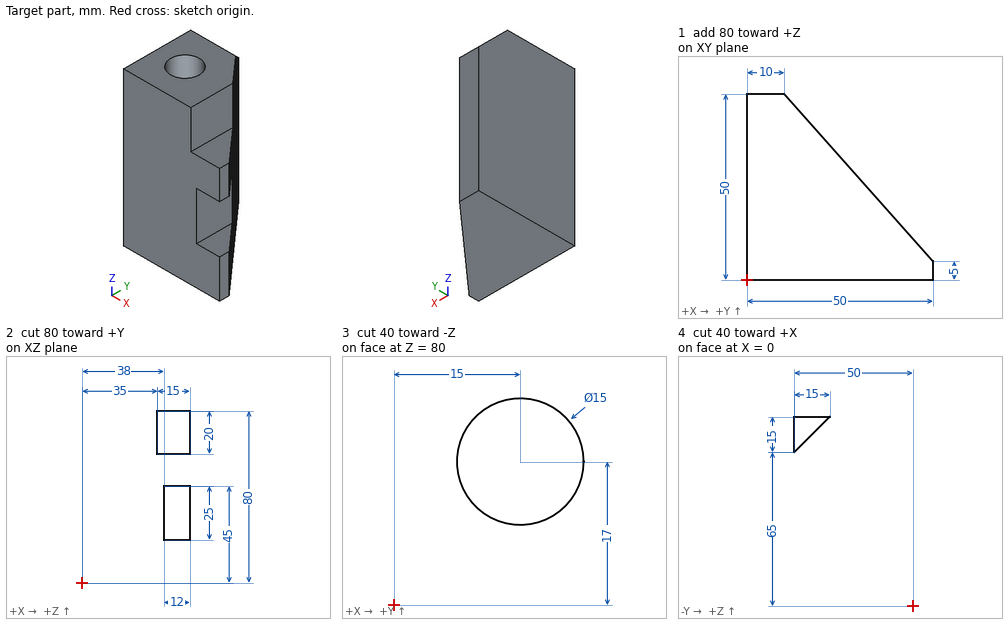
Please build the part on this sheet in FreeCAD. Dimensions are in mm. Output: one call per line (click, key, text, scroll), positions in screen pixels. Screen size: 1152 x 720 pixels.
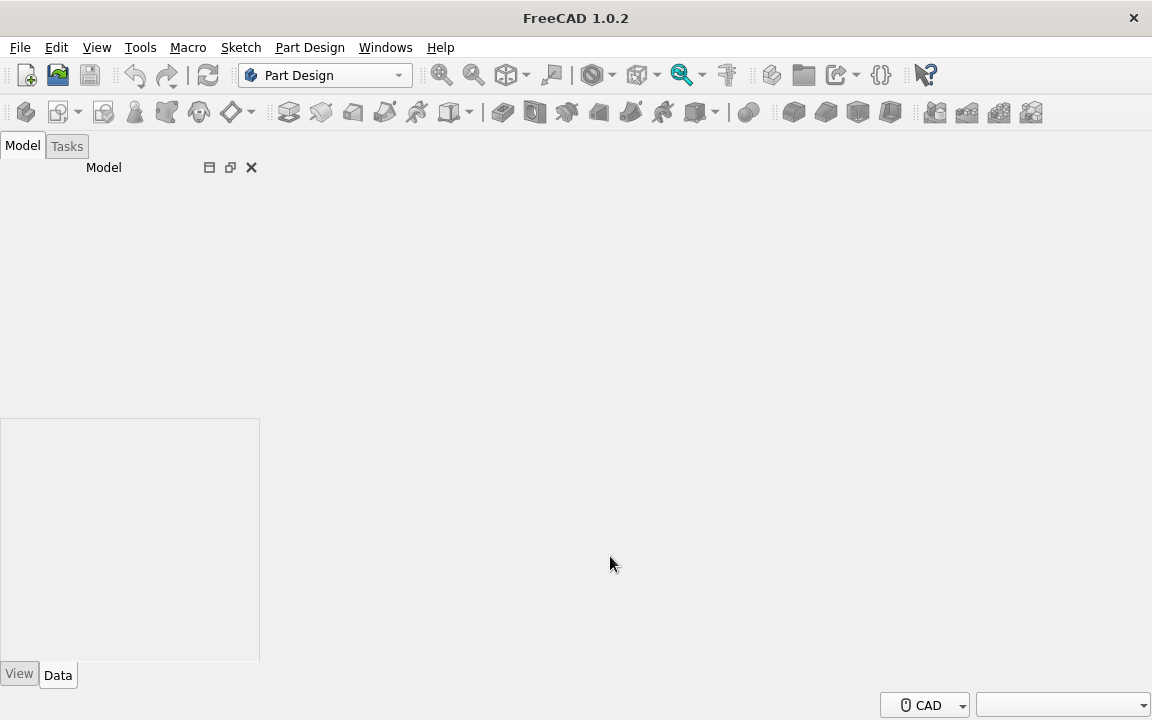
key(ctrl+n)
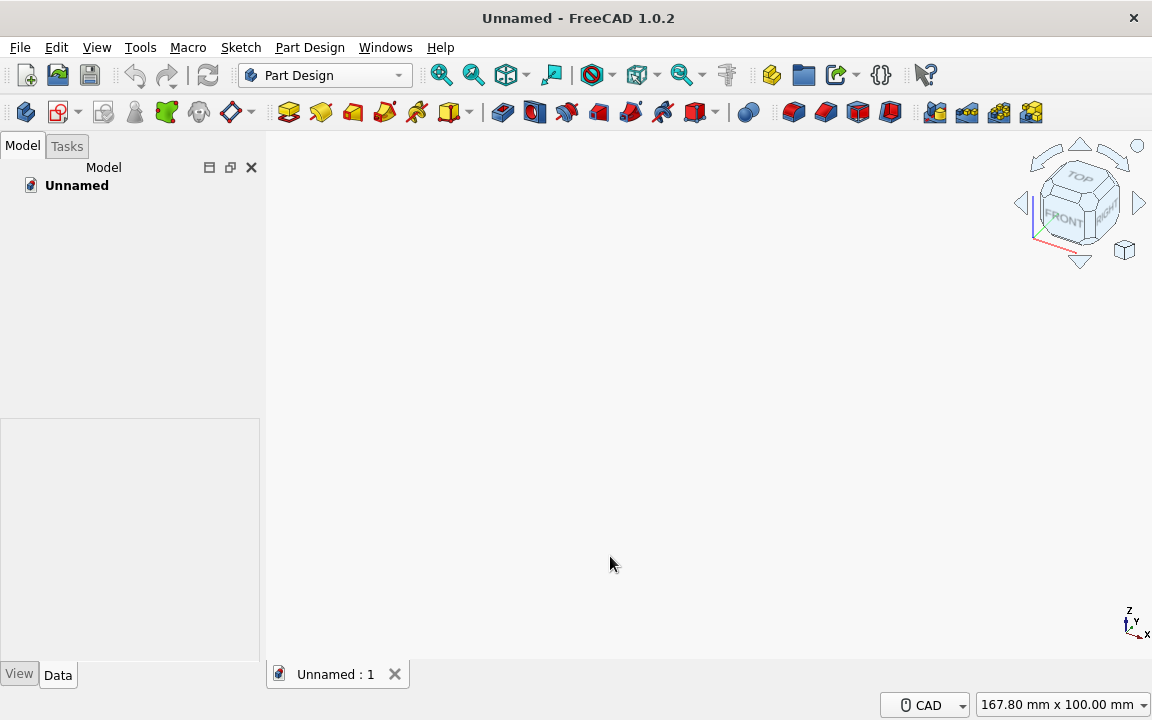
click(58, 112)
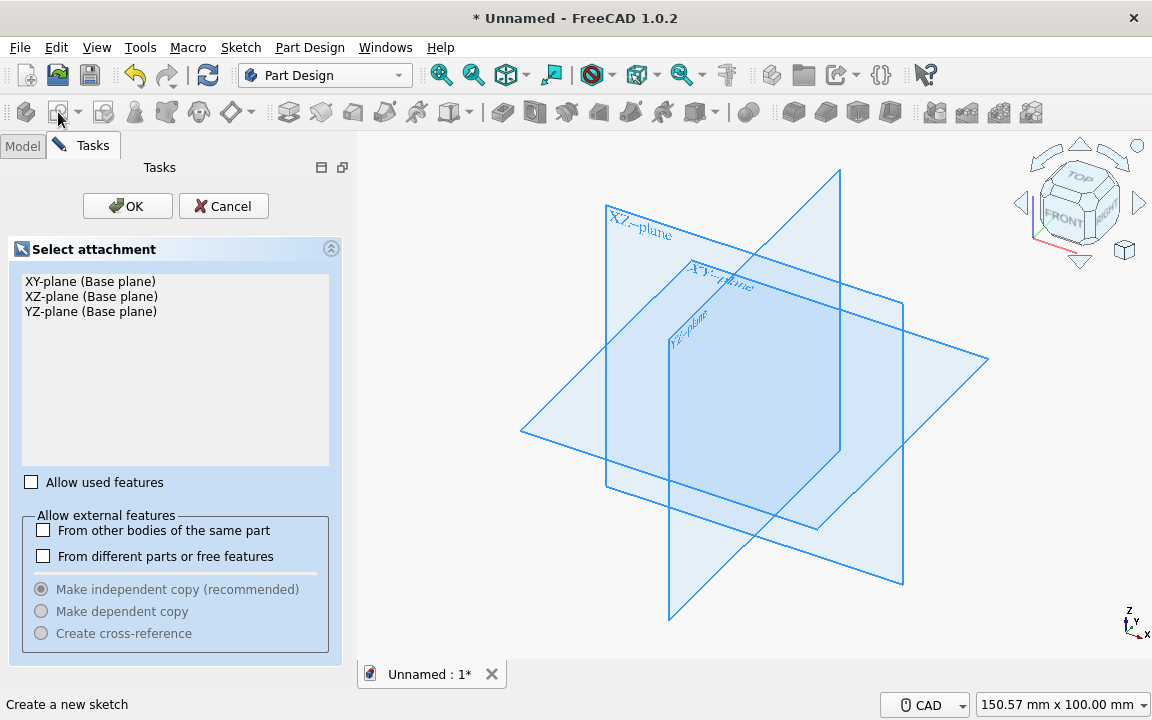
click(82, 282)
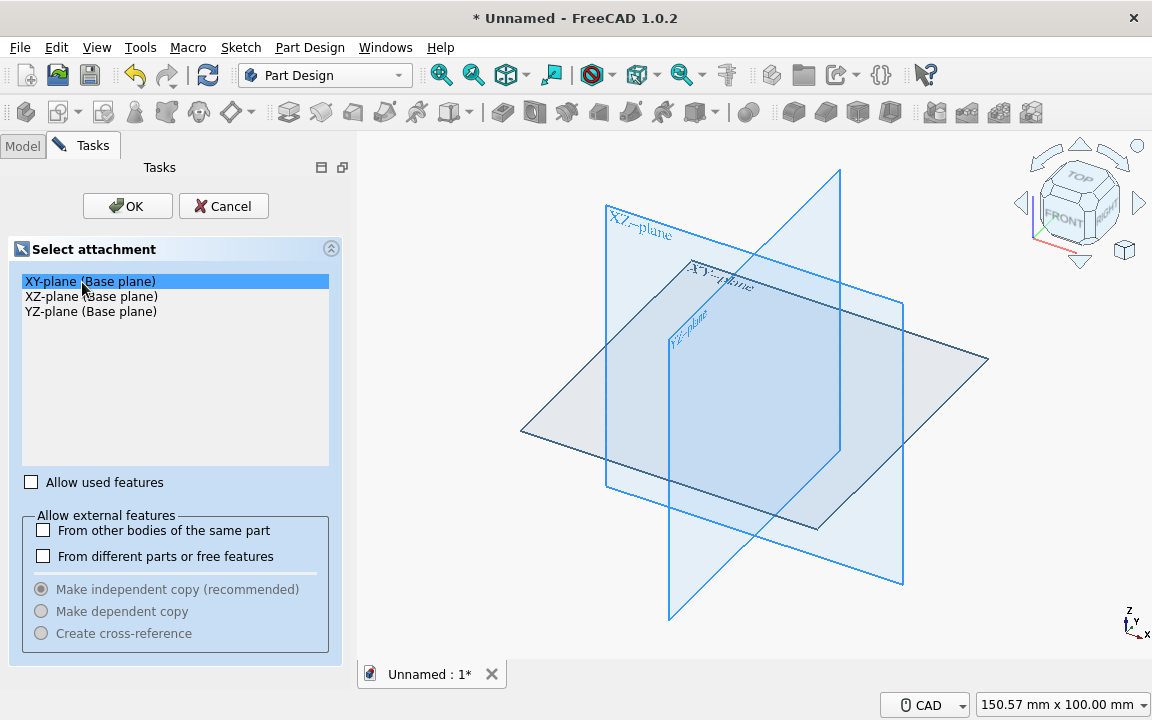
click(128, 206)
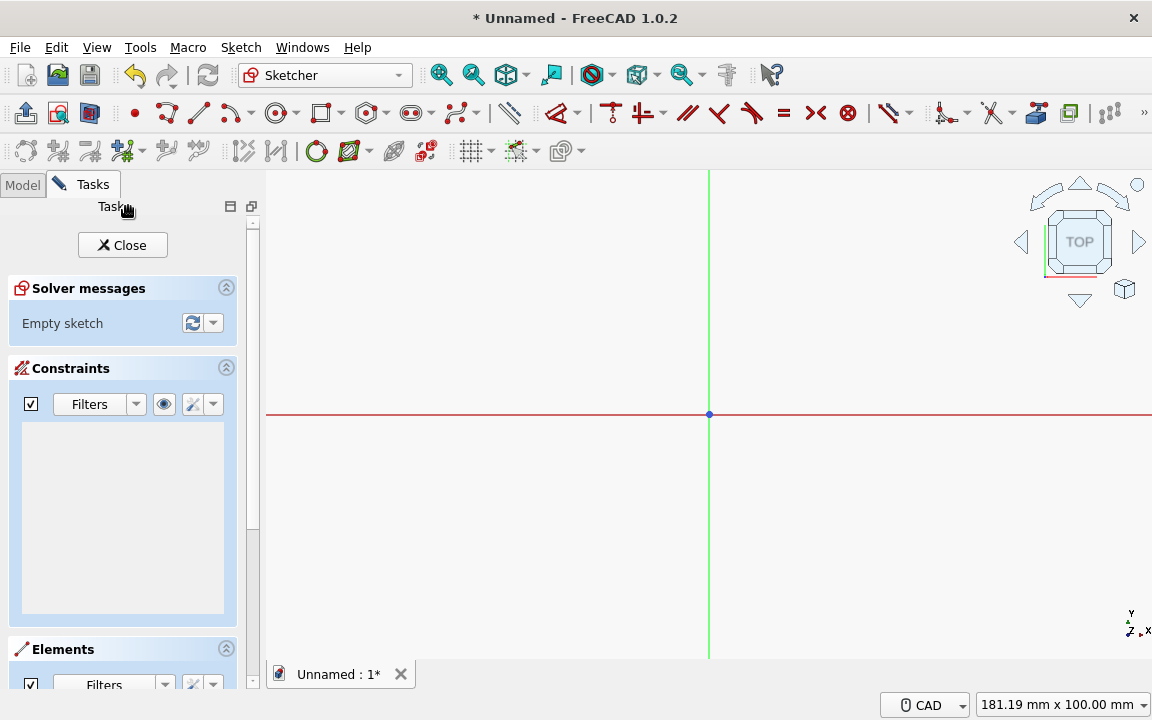
scroll(294, 631, down, 1)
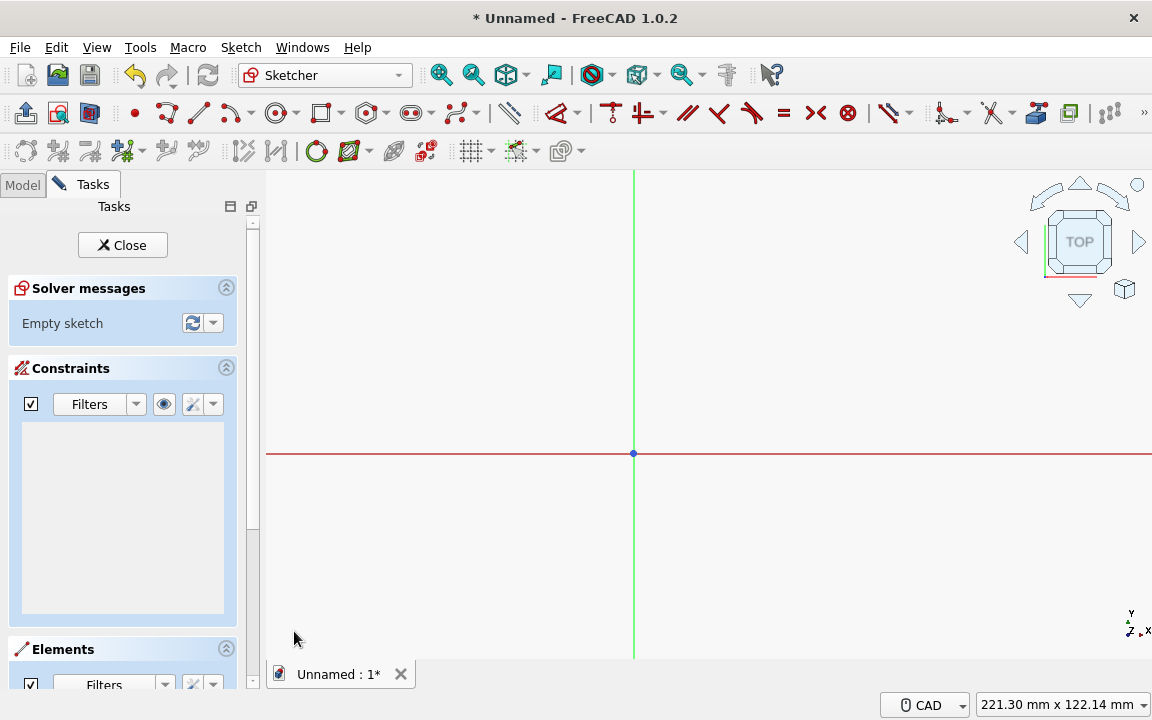
scroll(924, 230, up, 2)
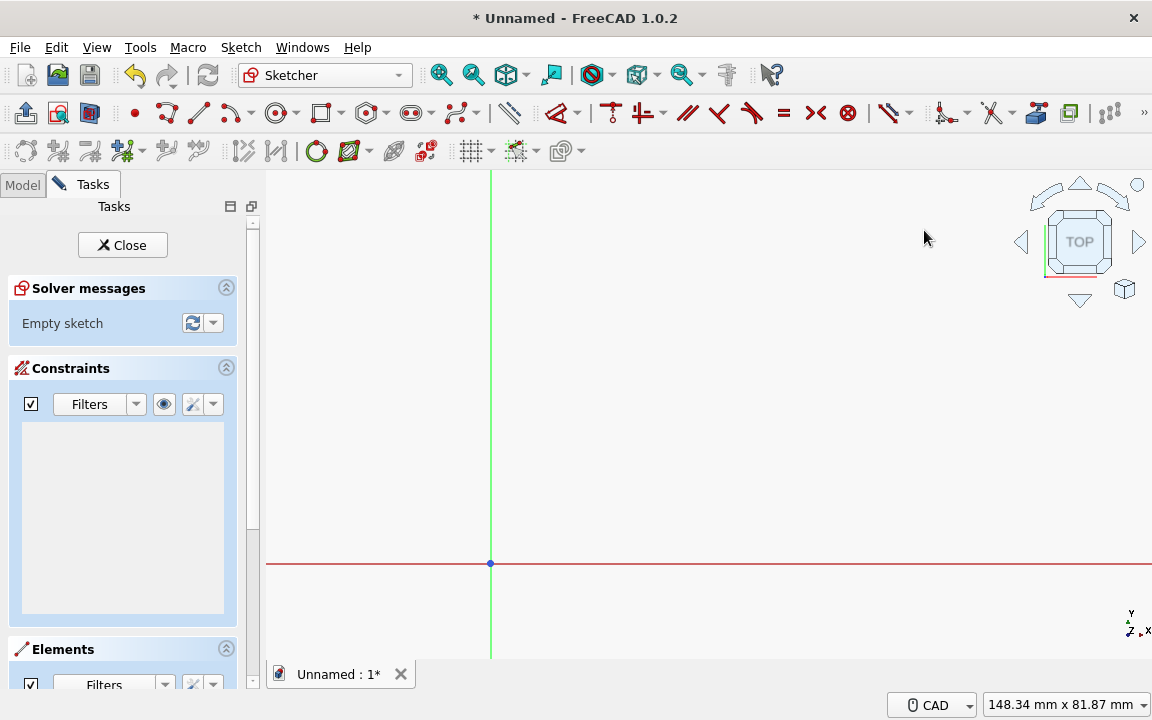
click(168, 114)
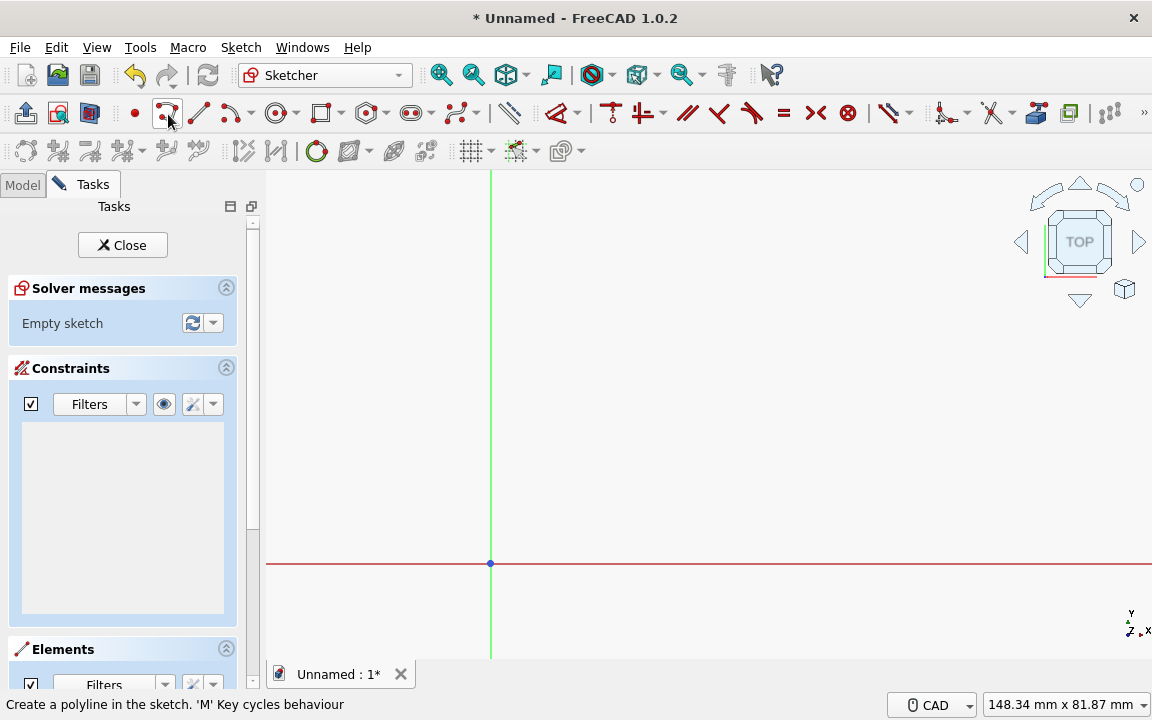
click(491, 564)
click(789, 555)
click(789, 534)
click(550, 265)
click(500, 265)
click(491, 564)
key(Escape)
key(Escape)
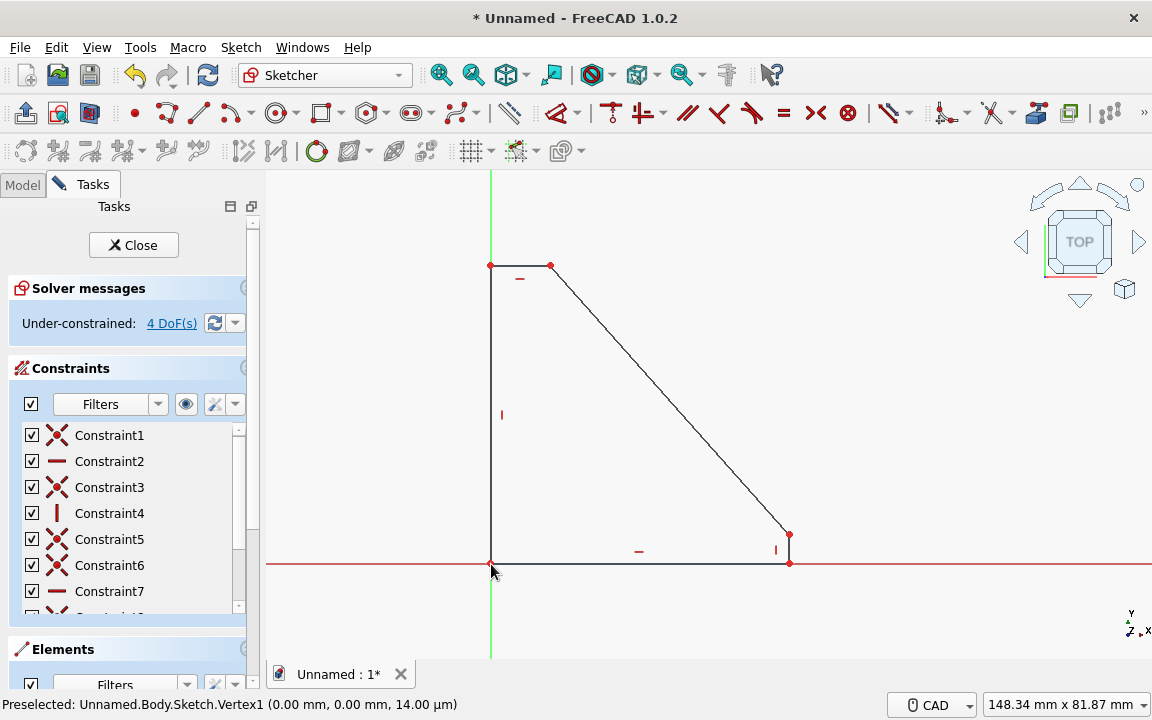
click(556, 114)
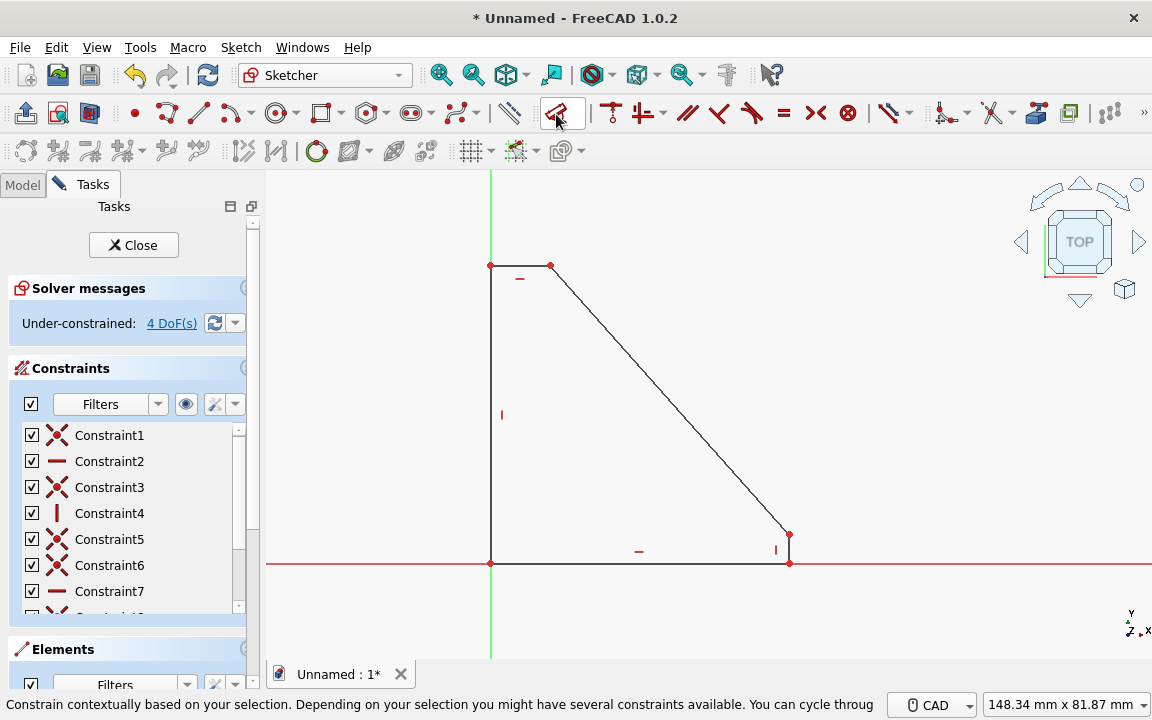
scroll(789, 552, up, 2)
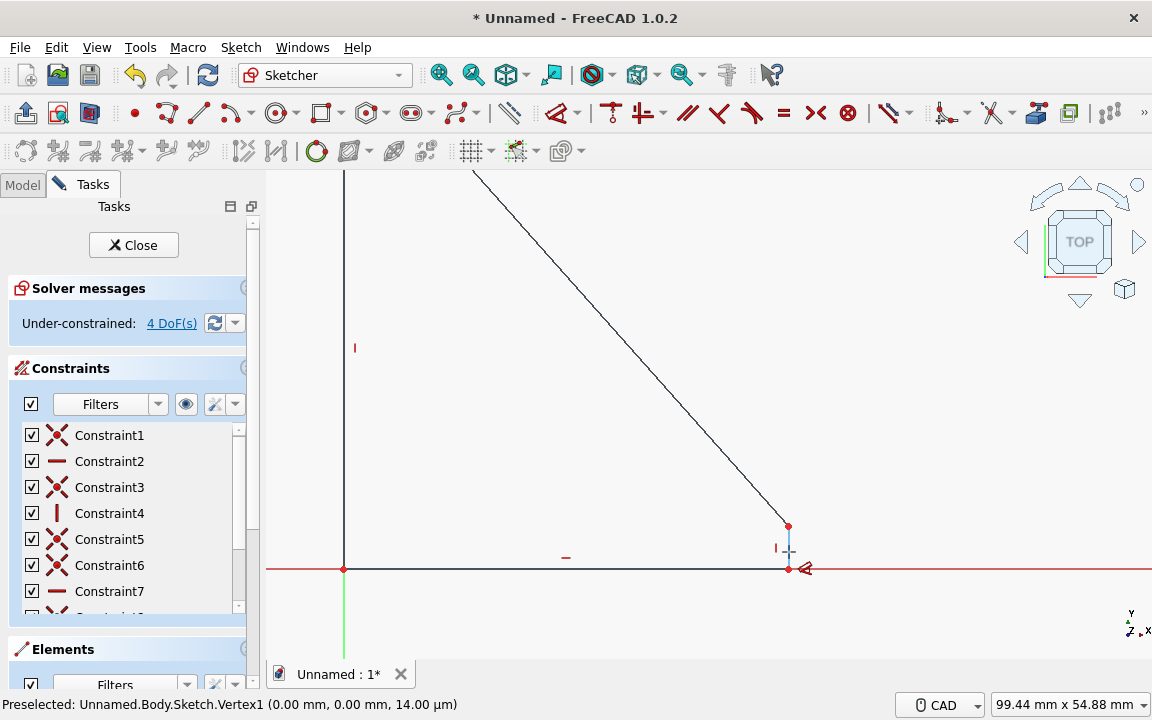
click(789, 552)
click(823, 548)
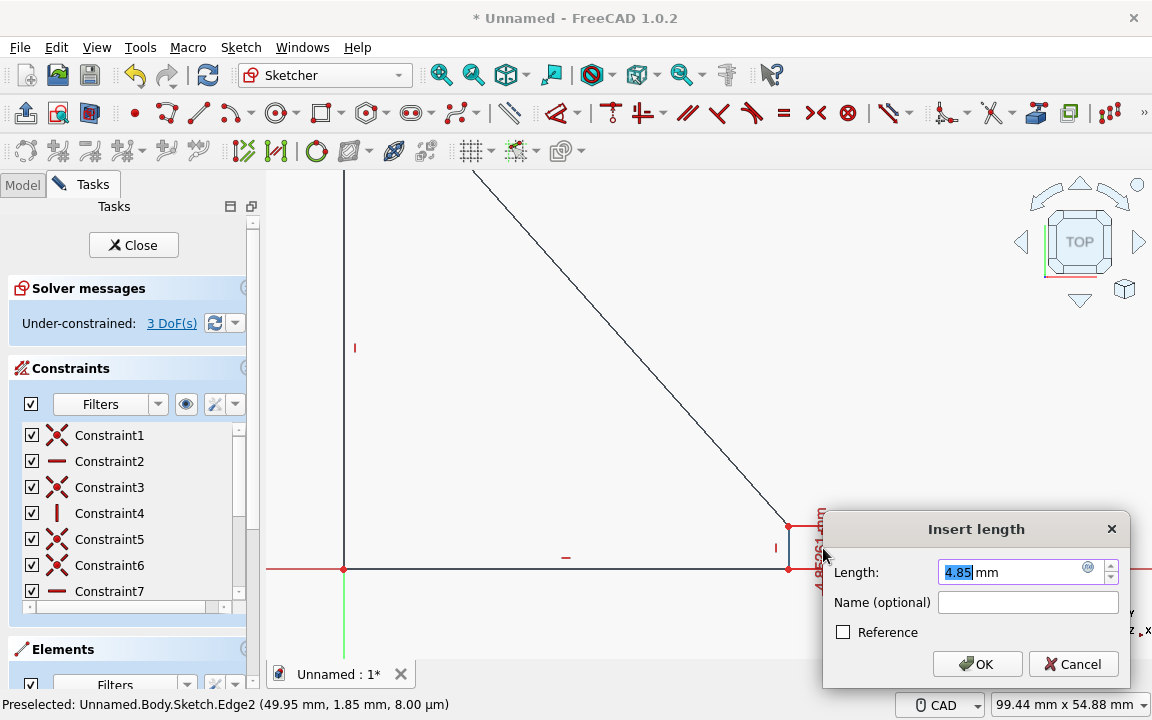
text(5)
key(Return)